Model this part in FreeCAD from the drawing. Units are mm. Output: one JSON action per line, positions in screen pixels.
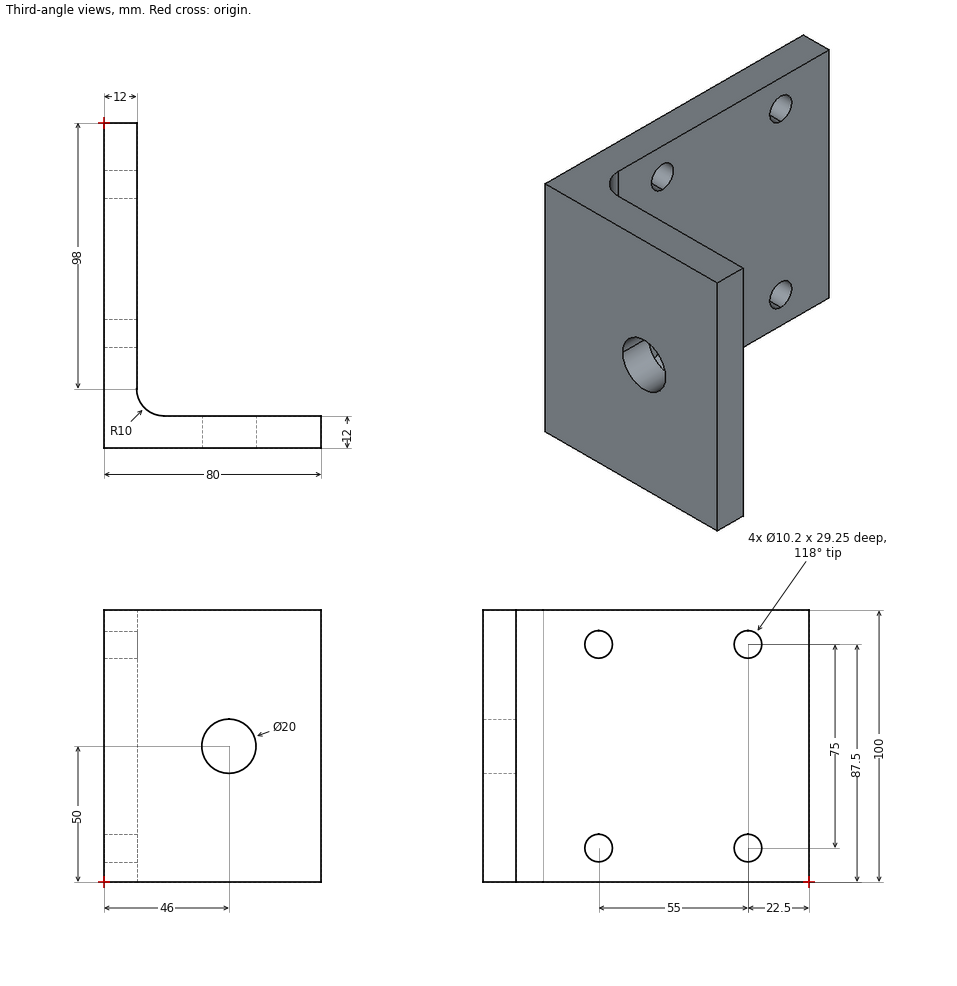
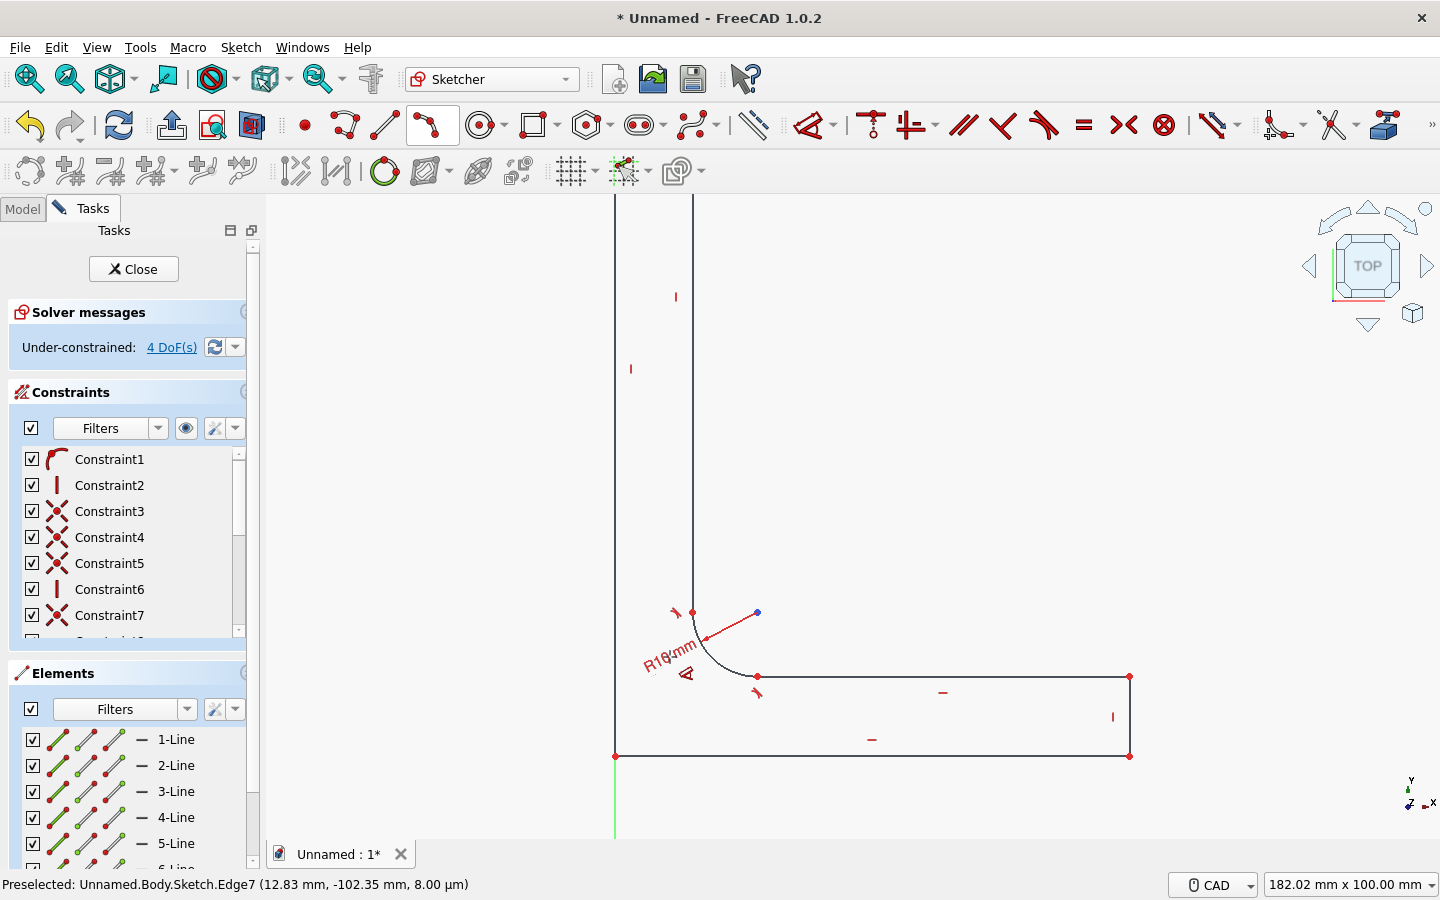
{"action": "left_click", "coordinate": [693, 423]}
{"action": "left_click", "coordinate": [659, 417]}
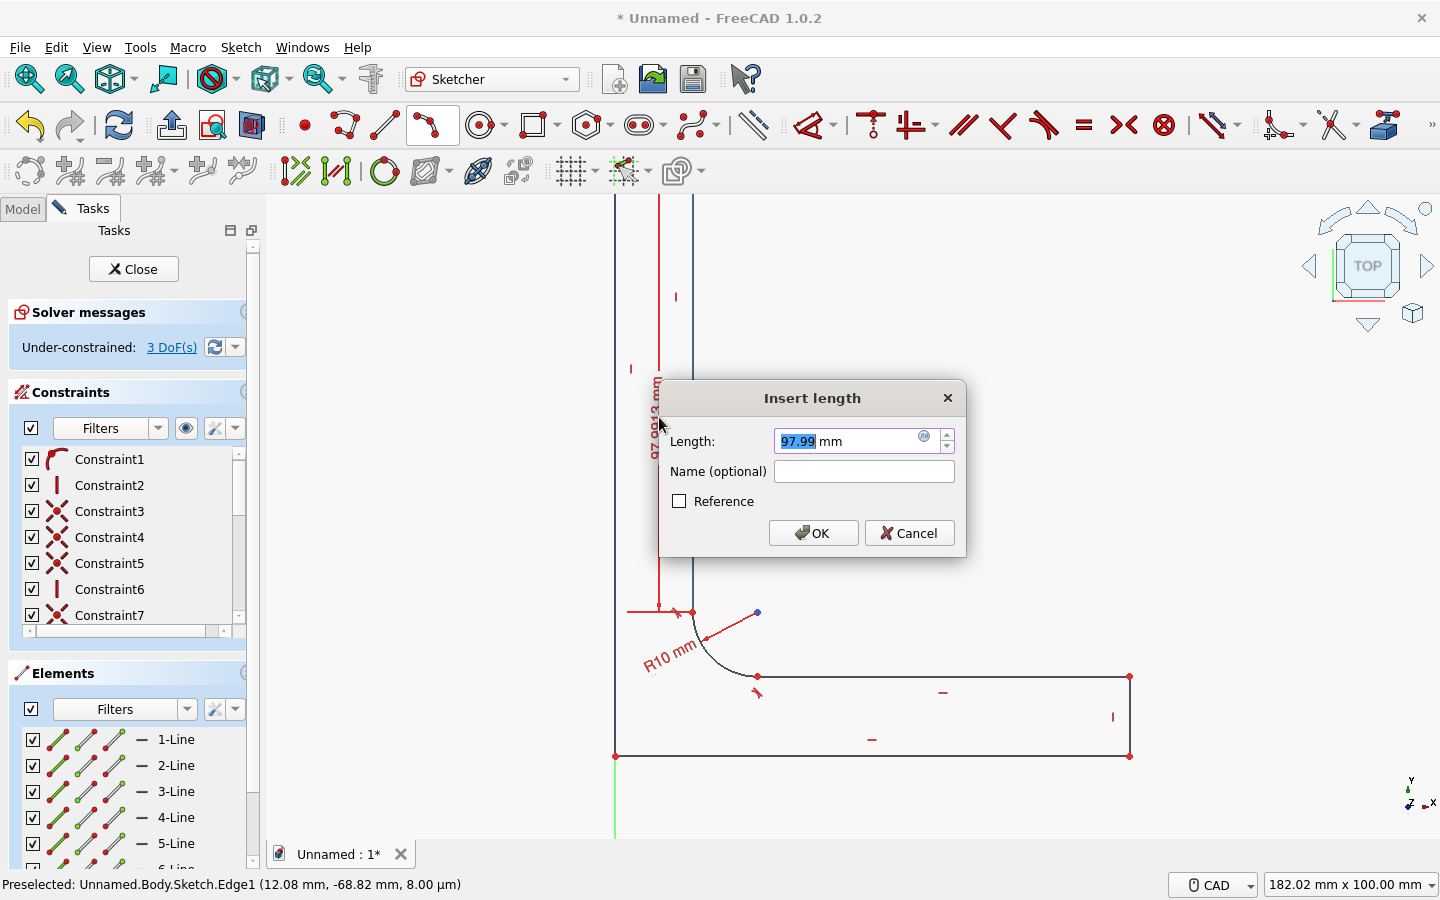
{"action": "type", "text": "98"}
{"action": "key", "text": "Return"}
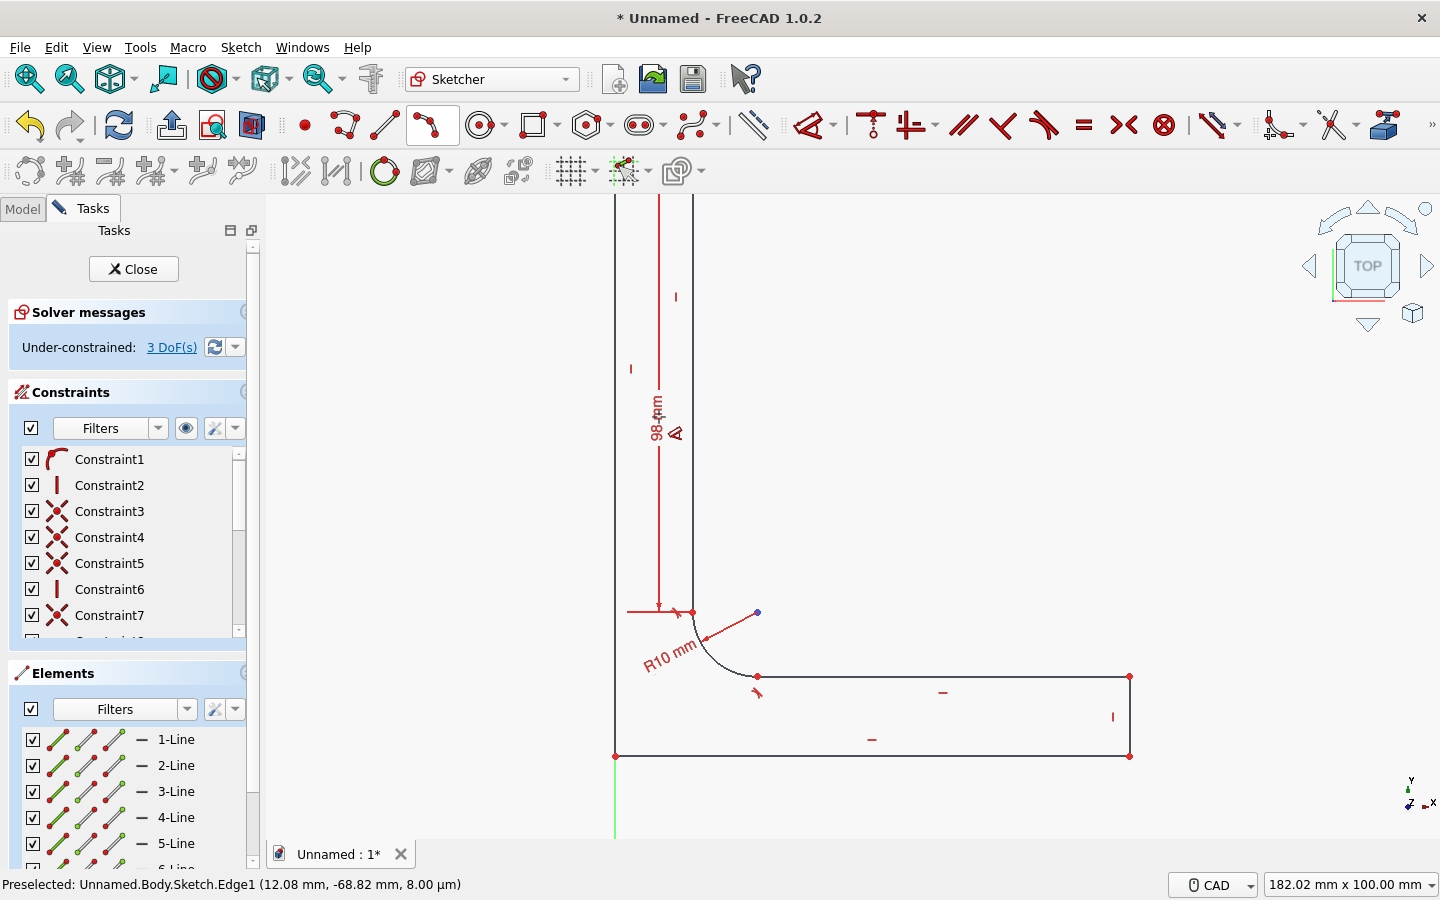
{"action": "scroll", "coordinate": [677, 698], "scroll_direction": "down", "scroll_amount": 3}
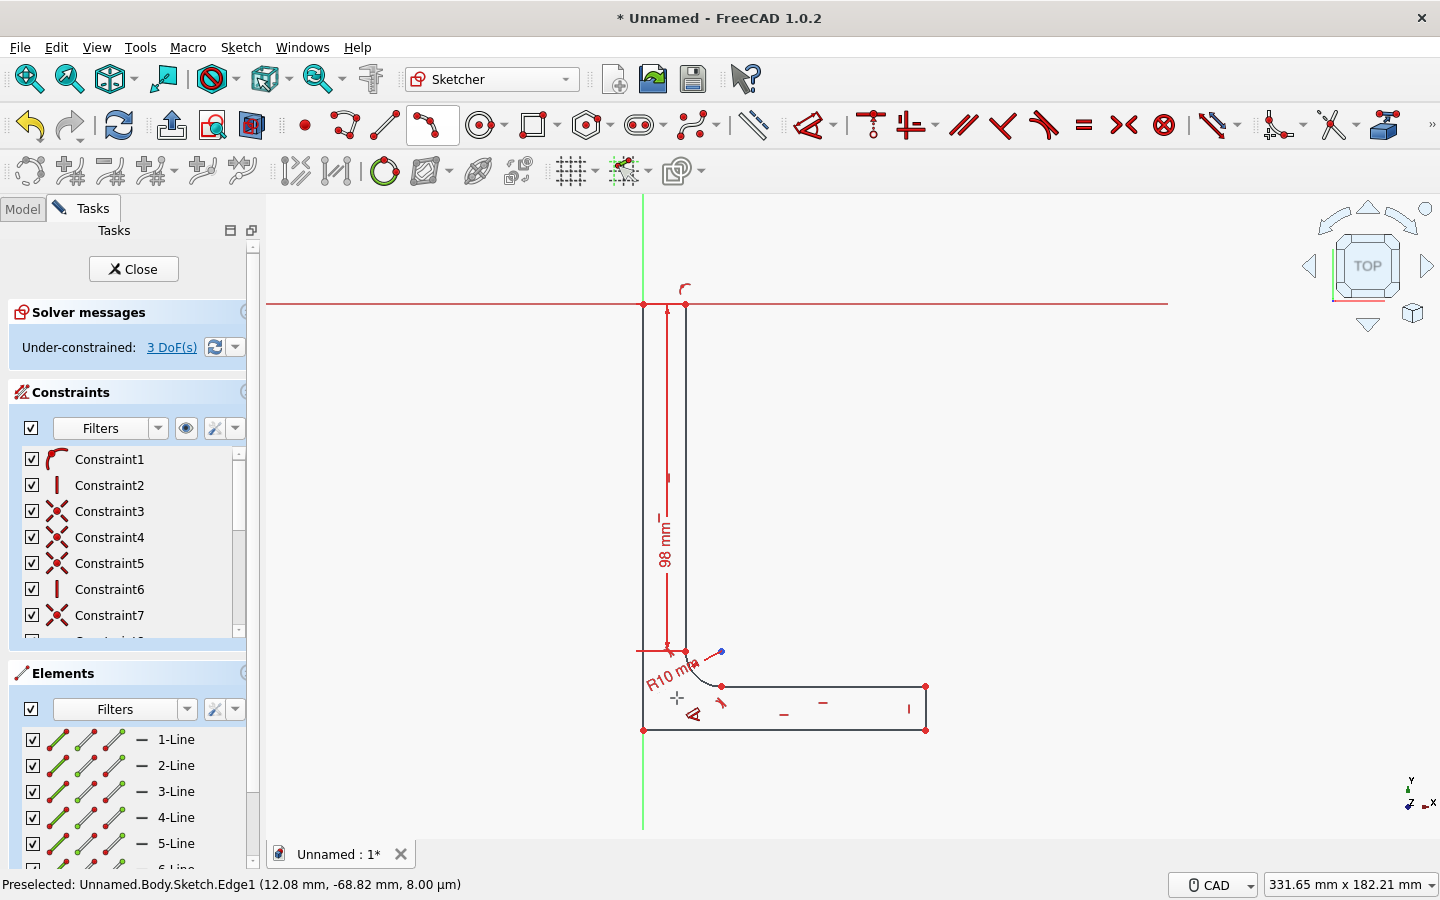
{"action": "left_click", "coordinate": [673, 304]}
{"action": "left_click", "coordinate": [665, 270]}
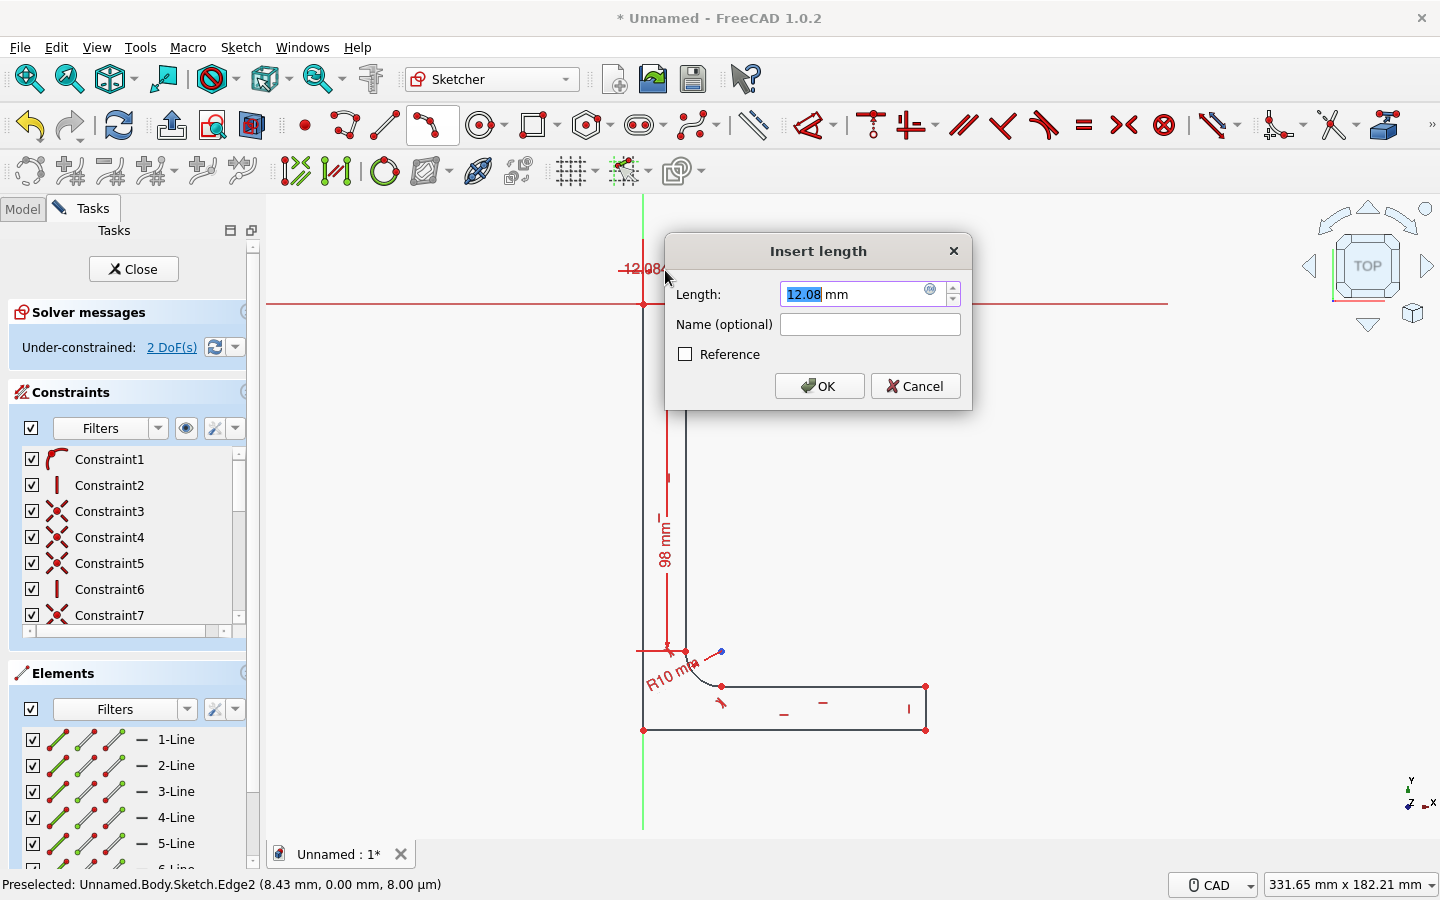
{"action": "type", "text": "12"}
{"action": "key", "text": "Return"}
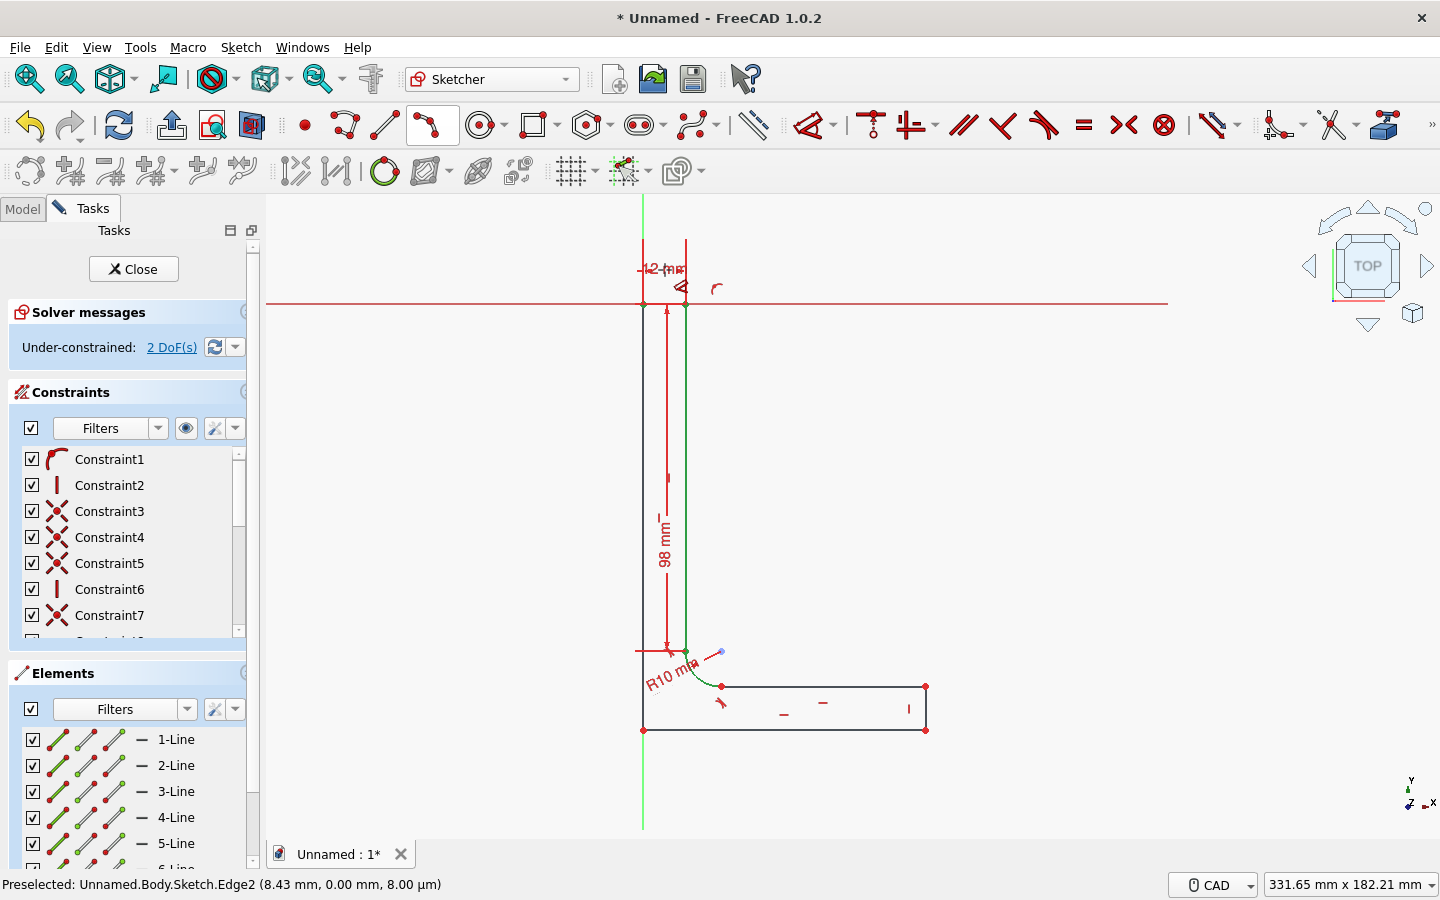
{"action": "left_click", "coordinate": [728, 730]}
{"action": "left_click", "coordinate": [784, 764]}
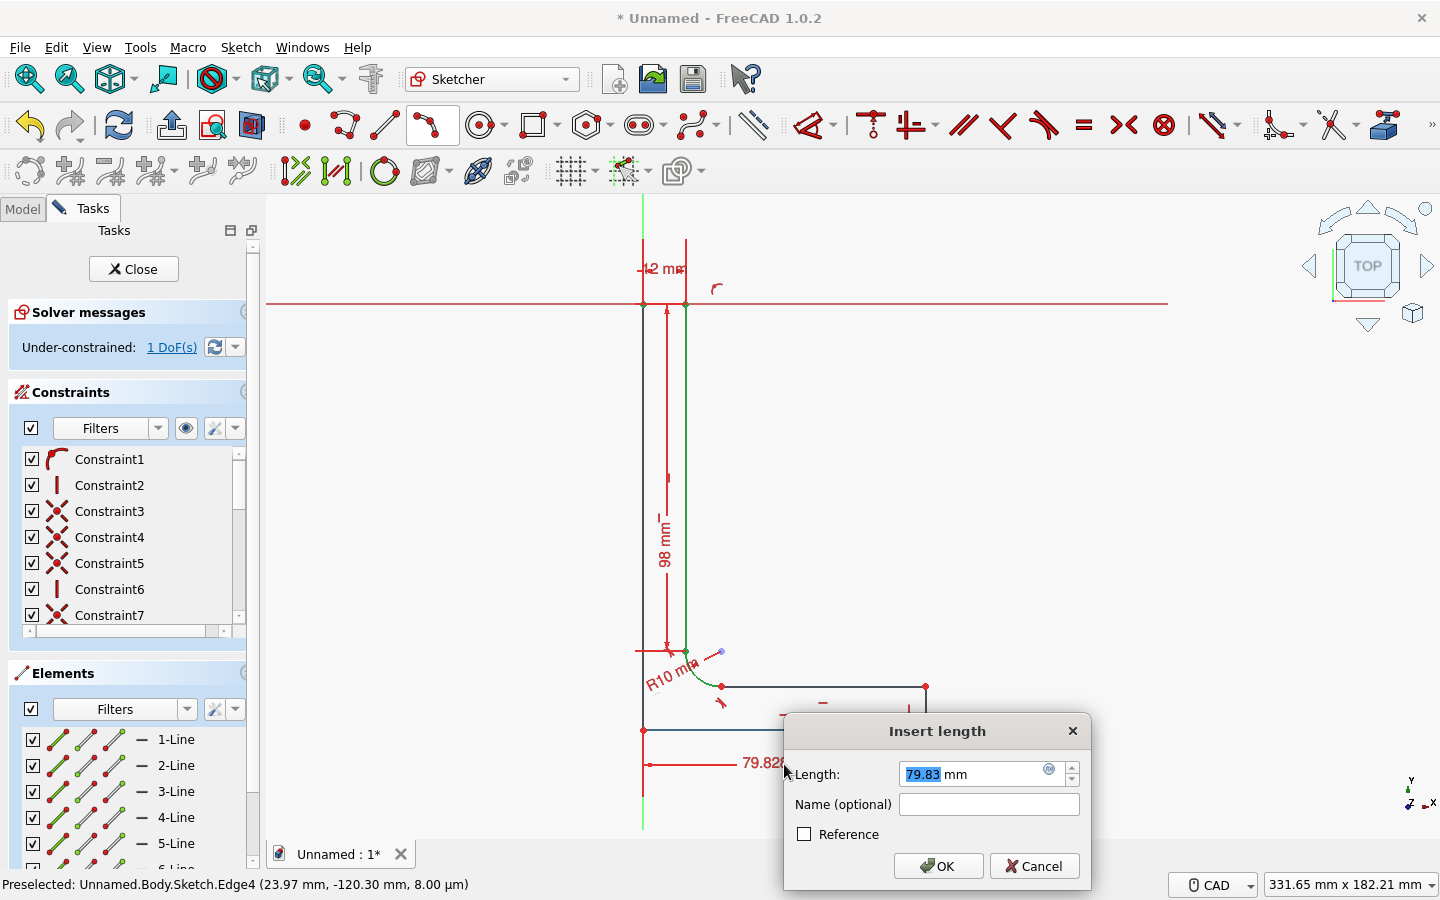
{"action": "type", "text": "80"}
{"action": "key", "text": "Return"}